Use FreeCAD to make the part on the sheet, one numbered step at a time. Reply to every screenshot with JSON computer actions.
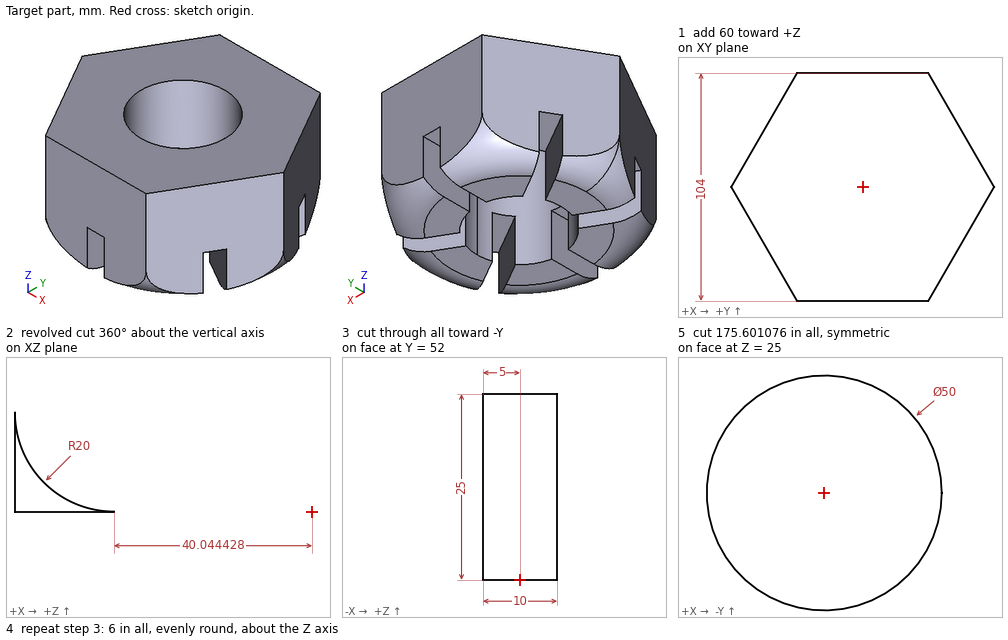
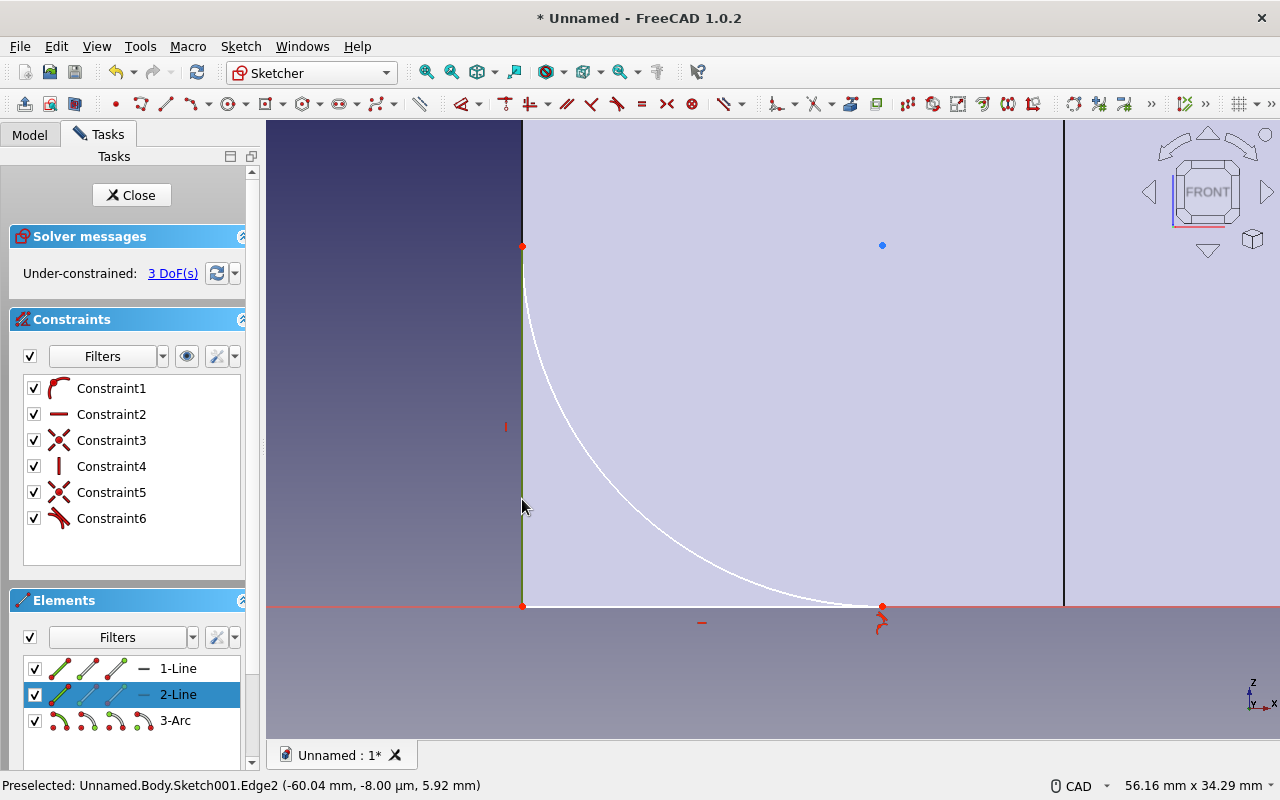
{"action": "left_click", "coordinate": [562, 410]}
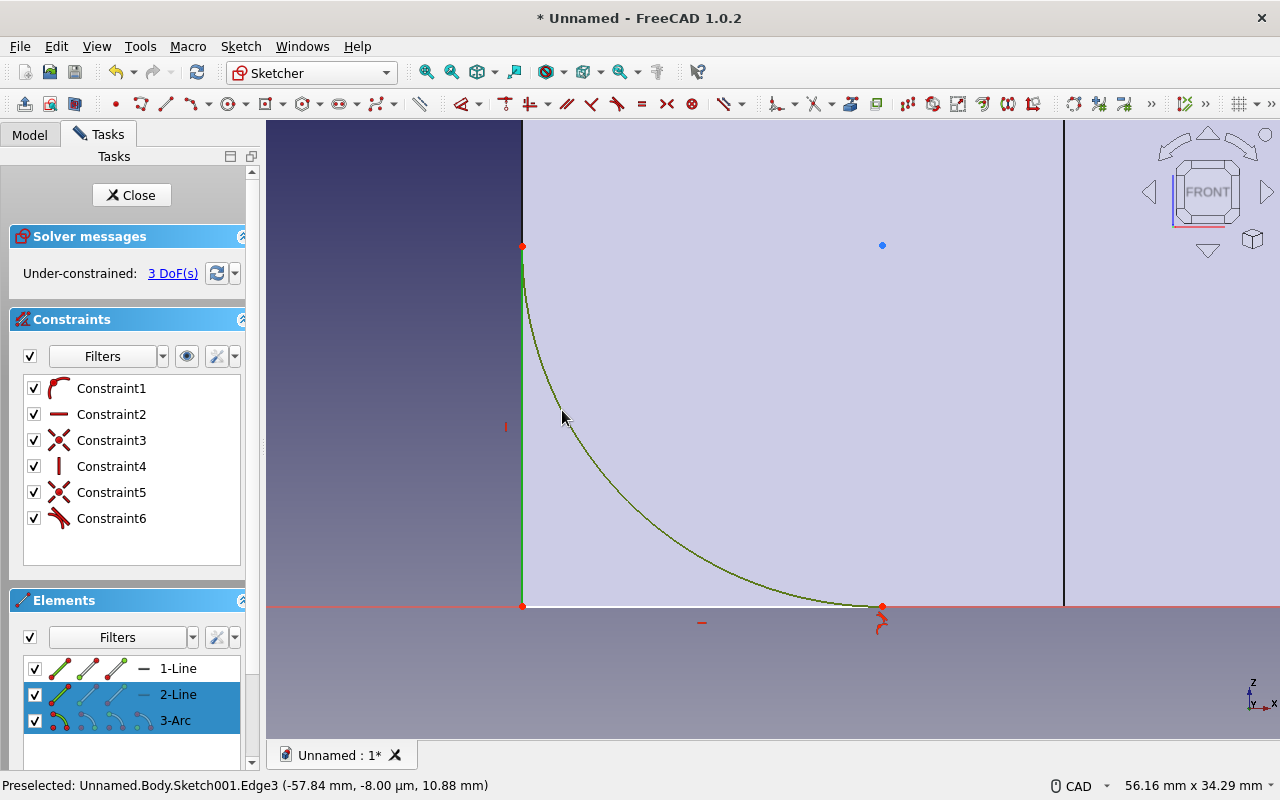
{"action": "key", "text": "t"}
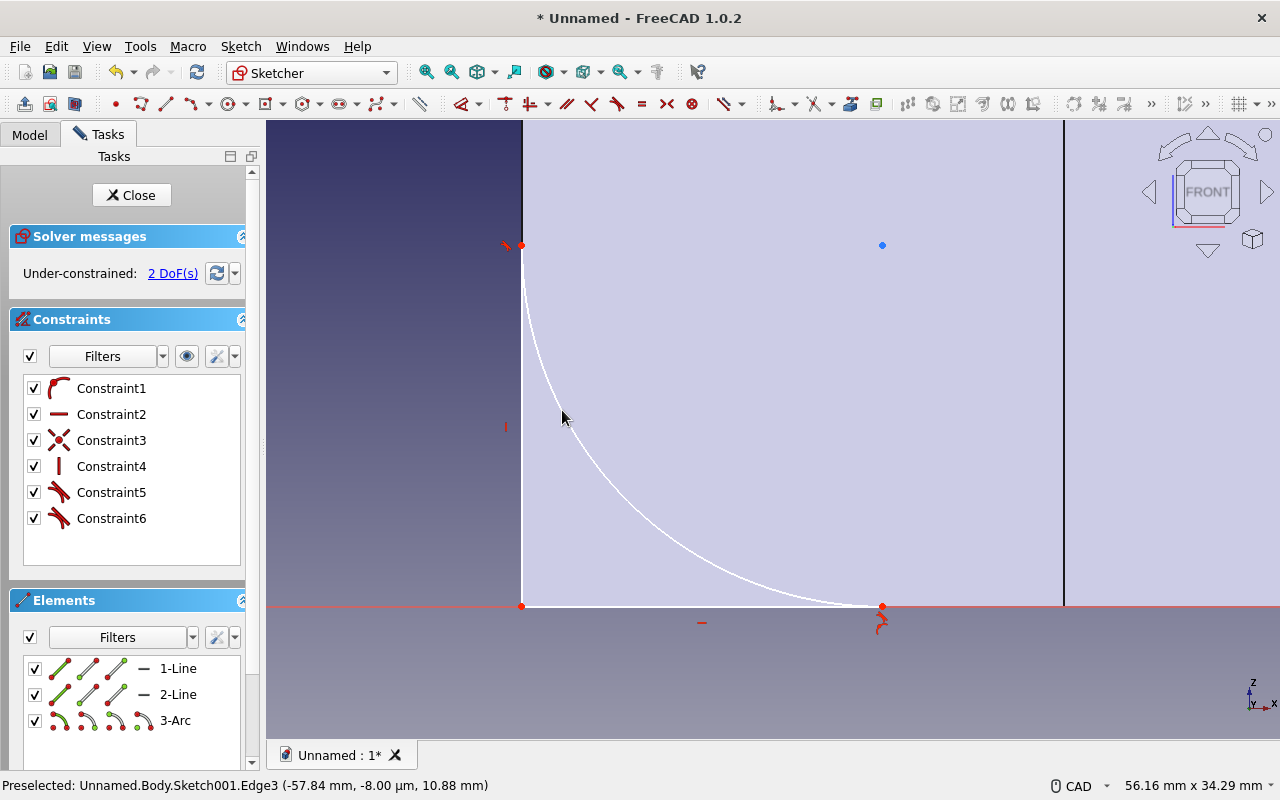
{"action": "key", "text": "d"}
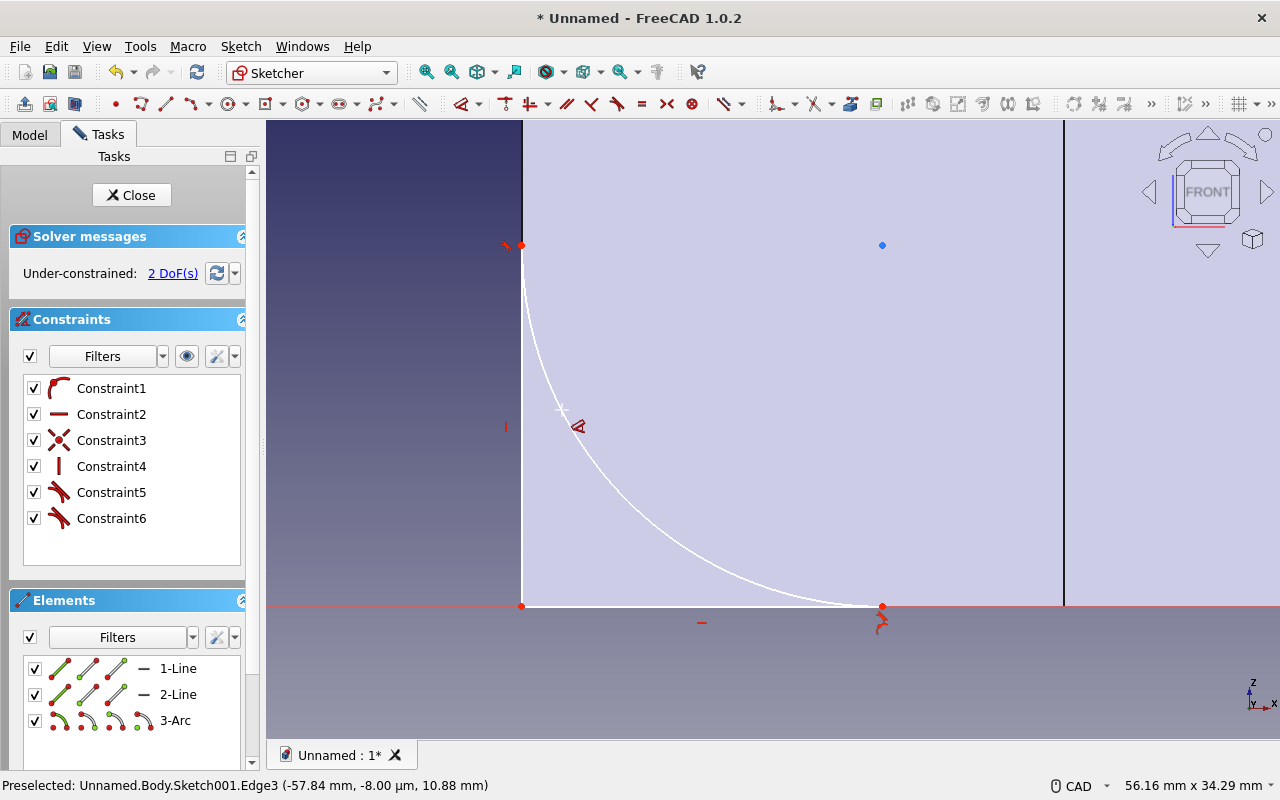
{"action": "left_click", "coordinate": [561, 410]}
{"action": "left_click", "coordinate": [490, 235]}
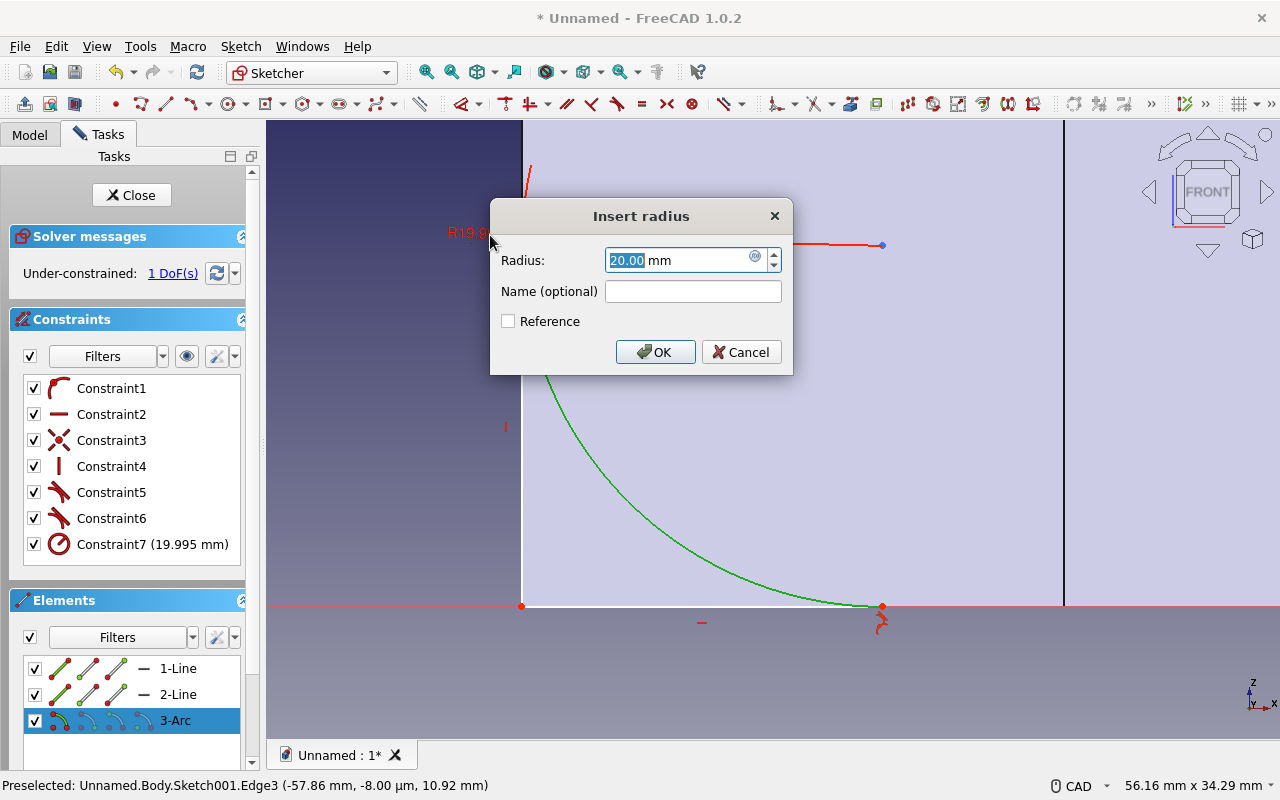
{"action": "type", "text": "20"}
{"action": "key", "text": "Return"}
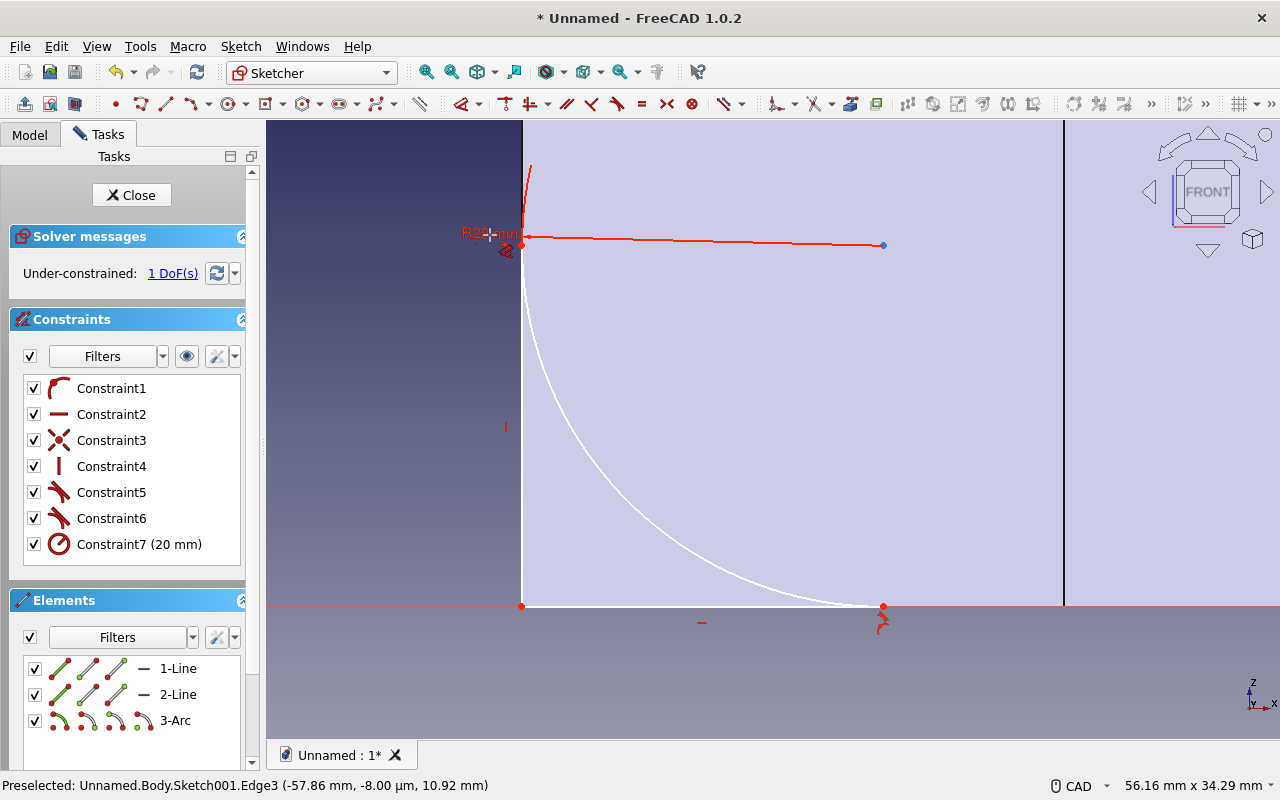
{"action": "left_click", "coordinate": [883, 607]}
{"action": "left_click", "coordinate": [999, 641]}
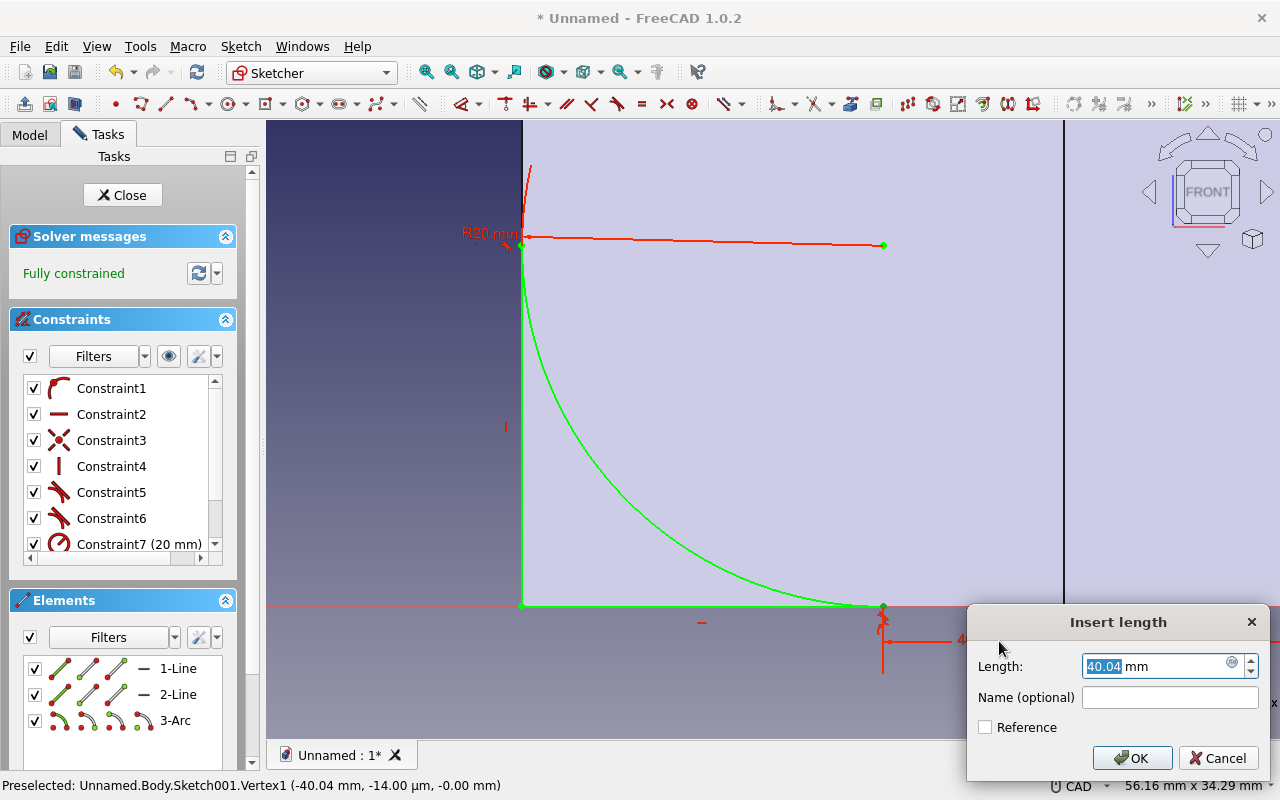
{"action": "type", "text": "40.044428"}
{"action": "key", "text": "Return"}
{"action": "key", "text": "Escape"}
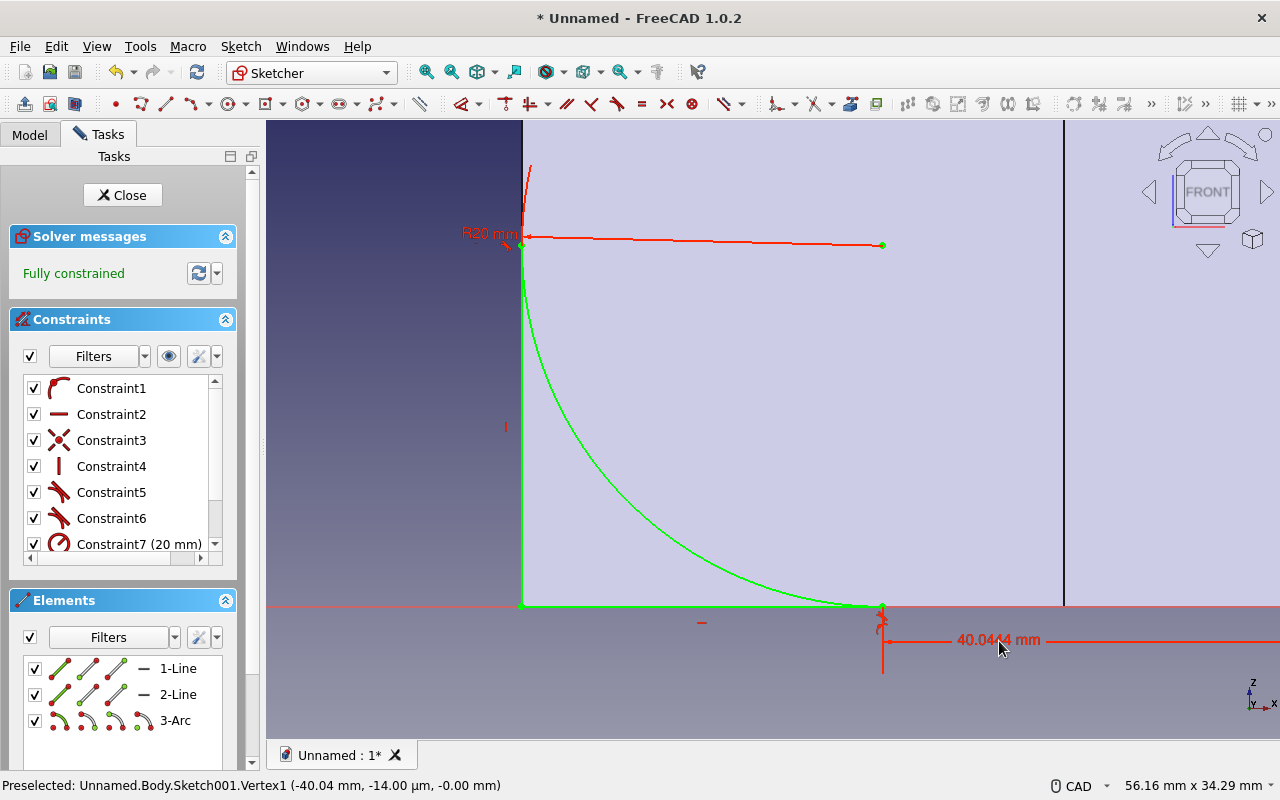
{"action": "left_click", "coordinate": [123, 195]}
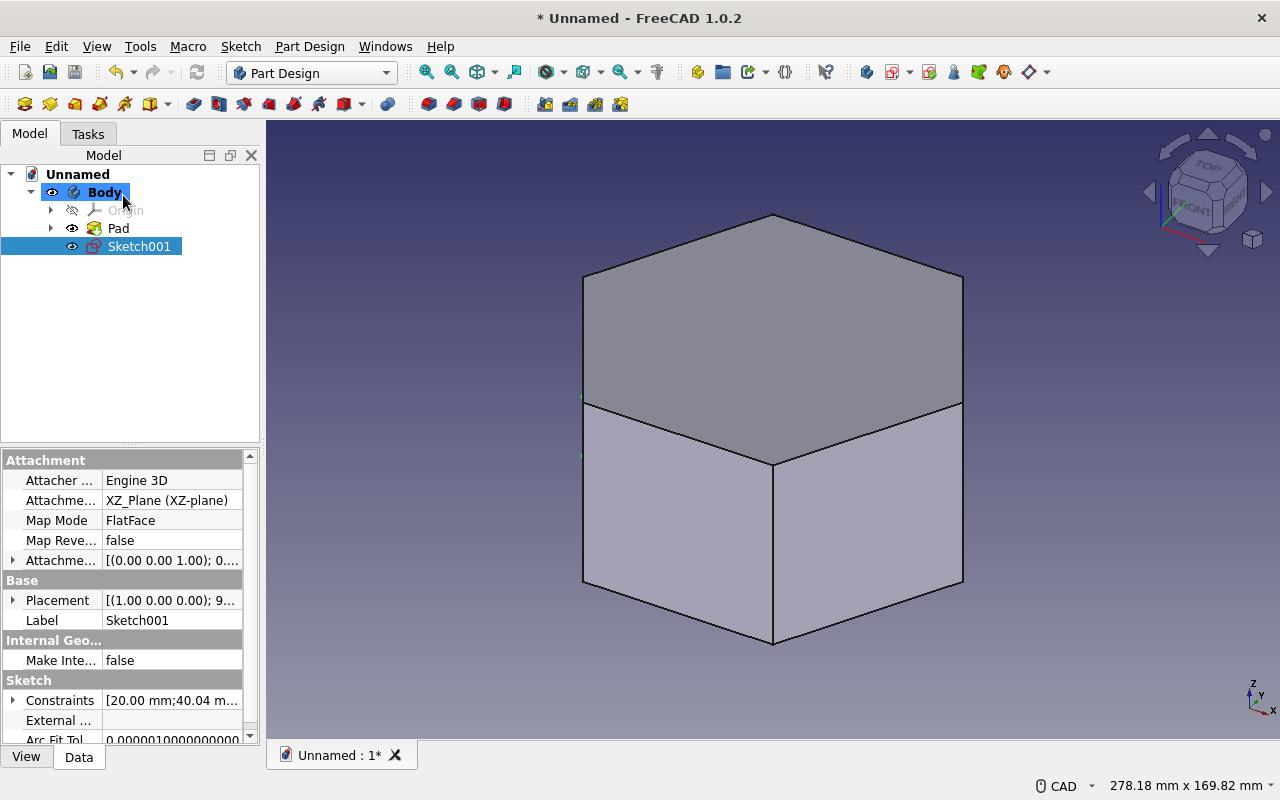
{"action": "left_click", "coordinate": [244, 104]}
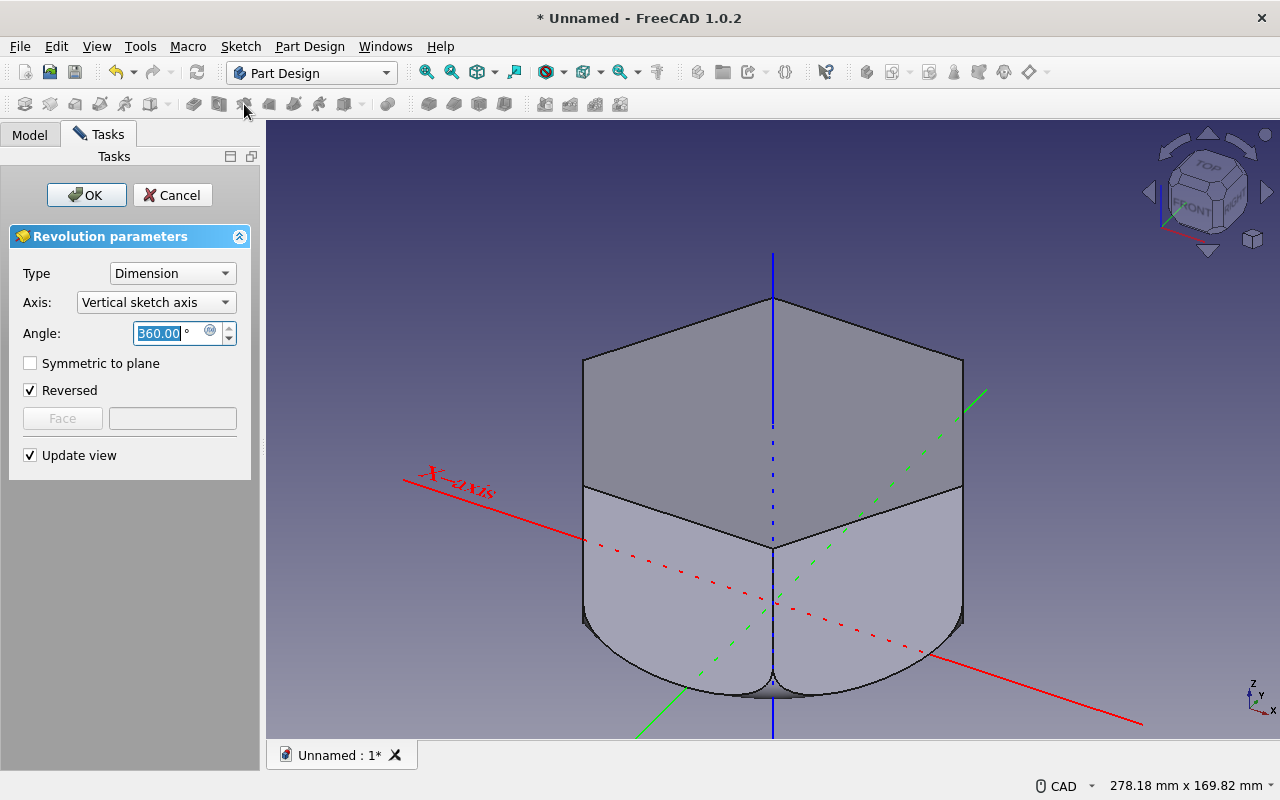
{"action": "left_click", "coordinate": [87, 195]}